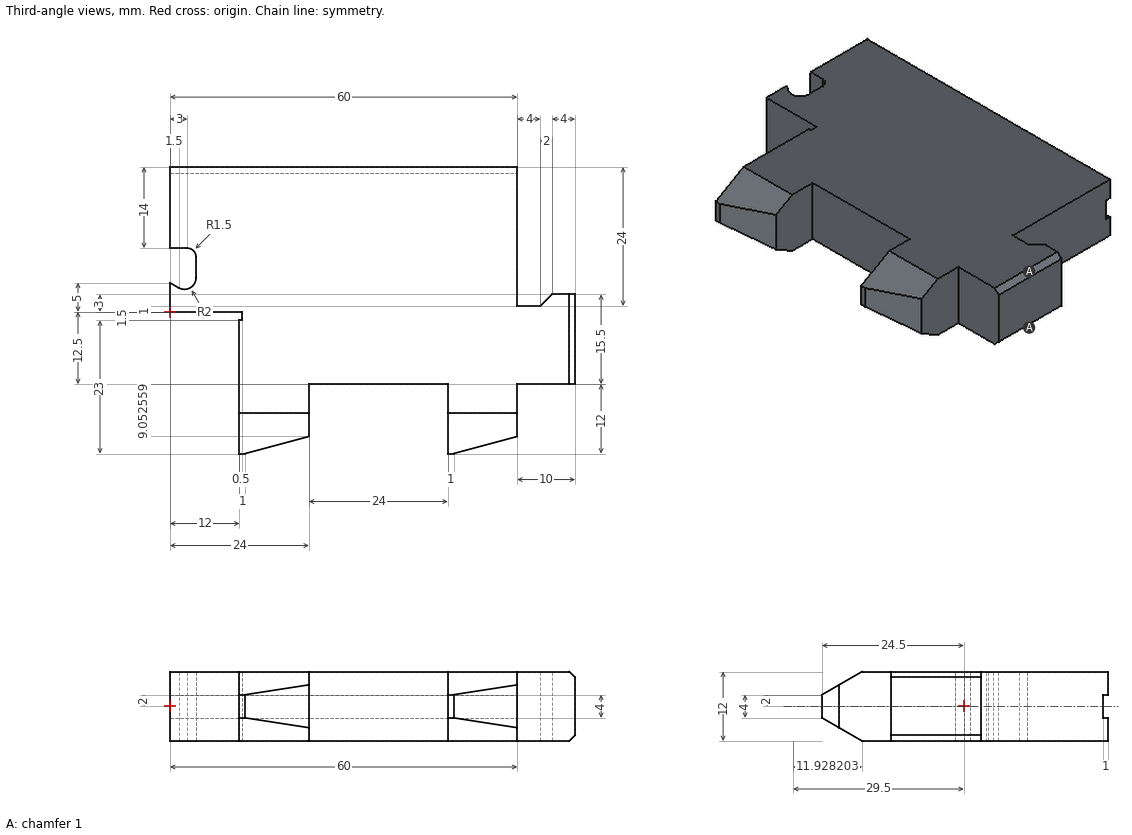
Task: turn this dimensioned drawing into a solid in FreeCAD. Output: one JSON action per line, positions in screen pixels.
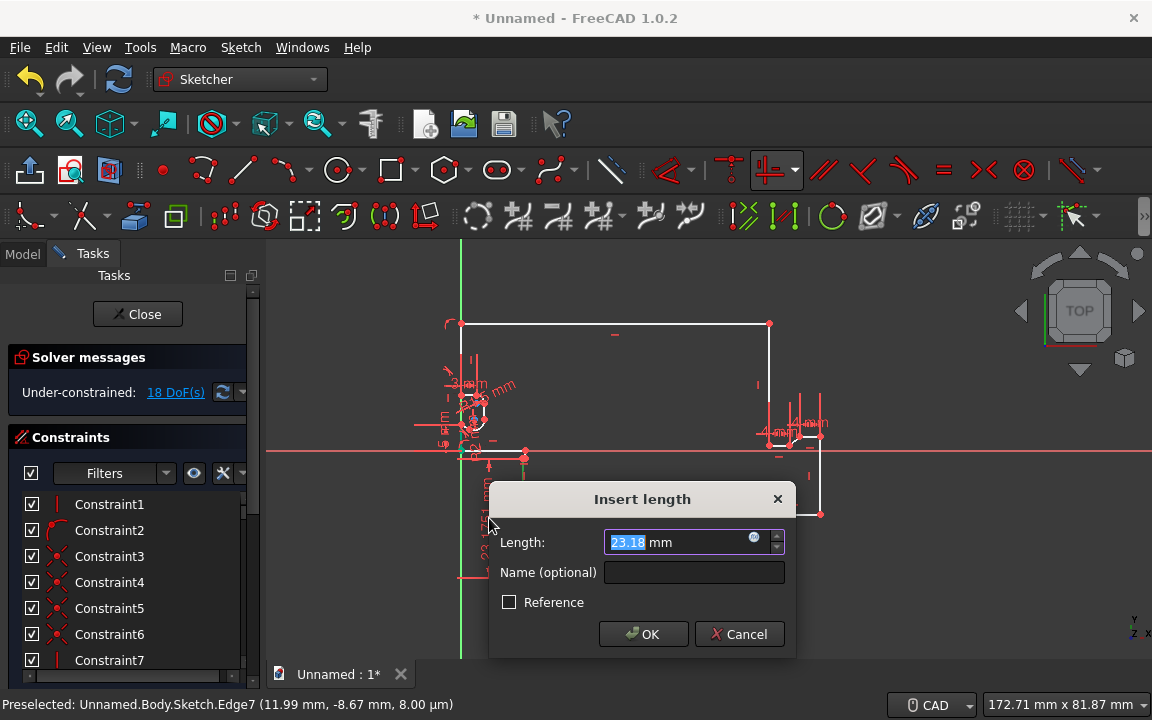
{"action": "type", "text": "23"}
{"action": "key", "text": "Return"}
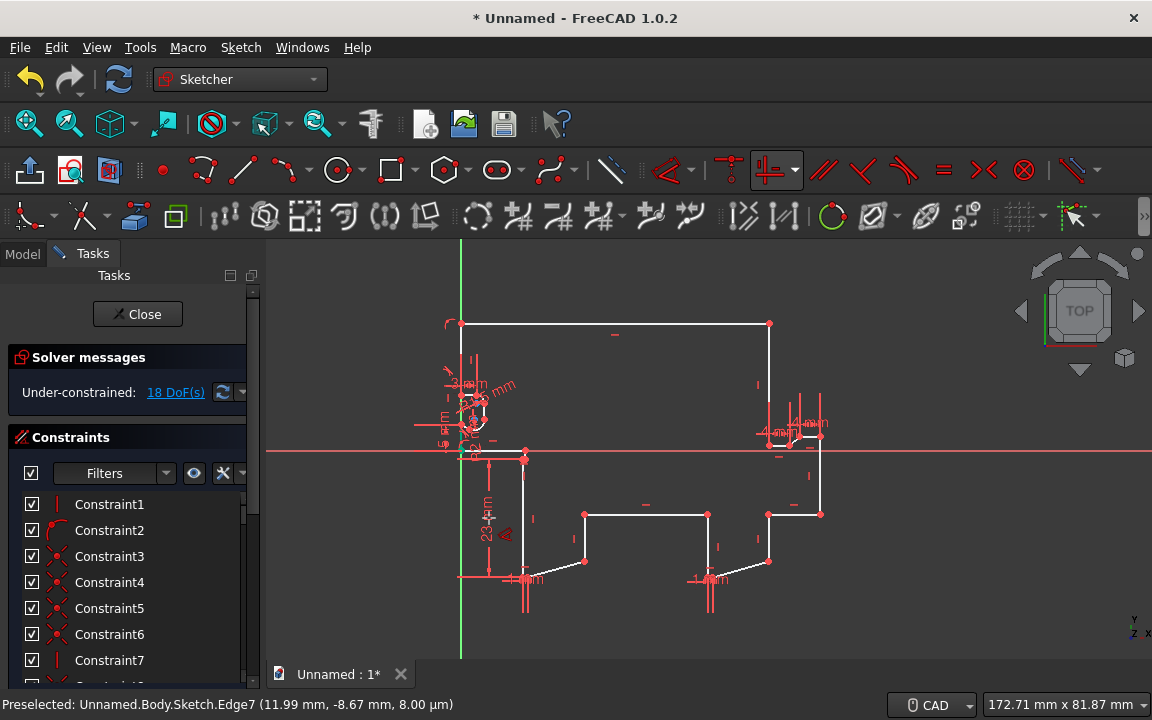
{"action": "left_click", "coordinate": [621, 515]}
{"action": "left_click", "coordinate": [646, 549]}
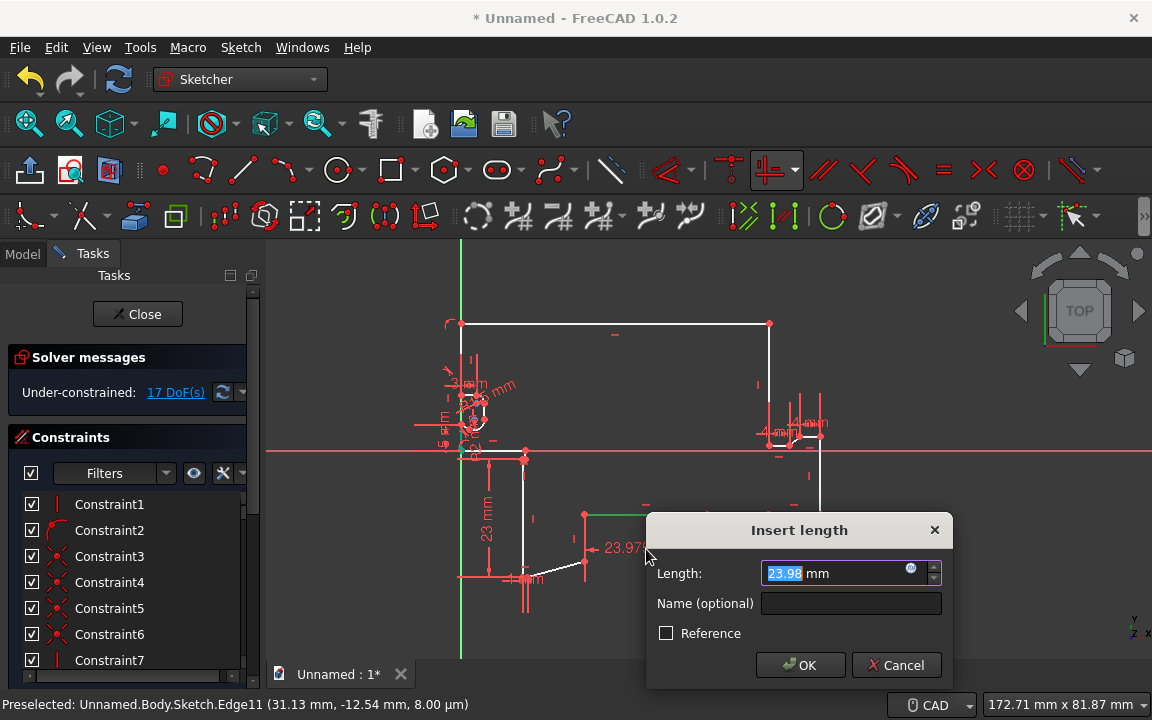
{"action": "type", "text": "24"}
{"action": "key", "text": "Return"}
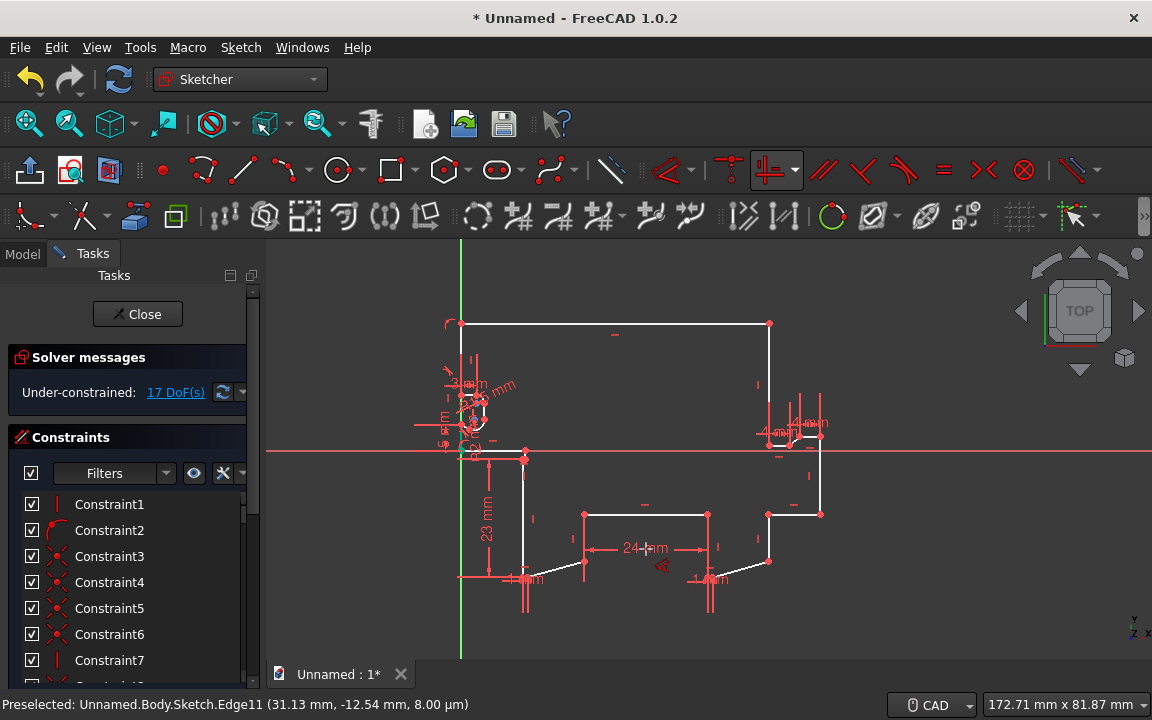
{"action": "left_click", "coordinate": [708, 534]}
{"action": "left_click", "coordinate": [742, 546]}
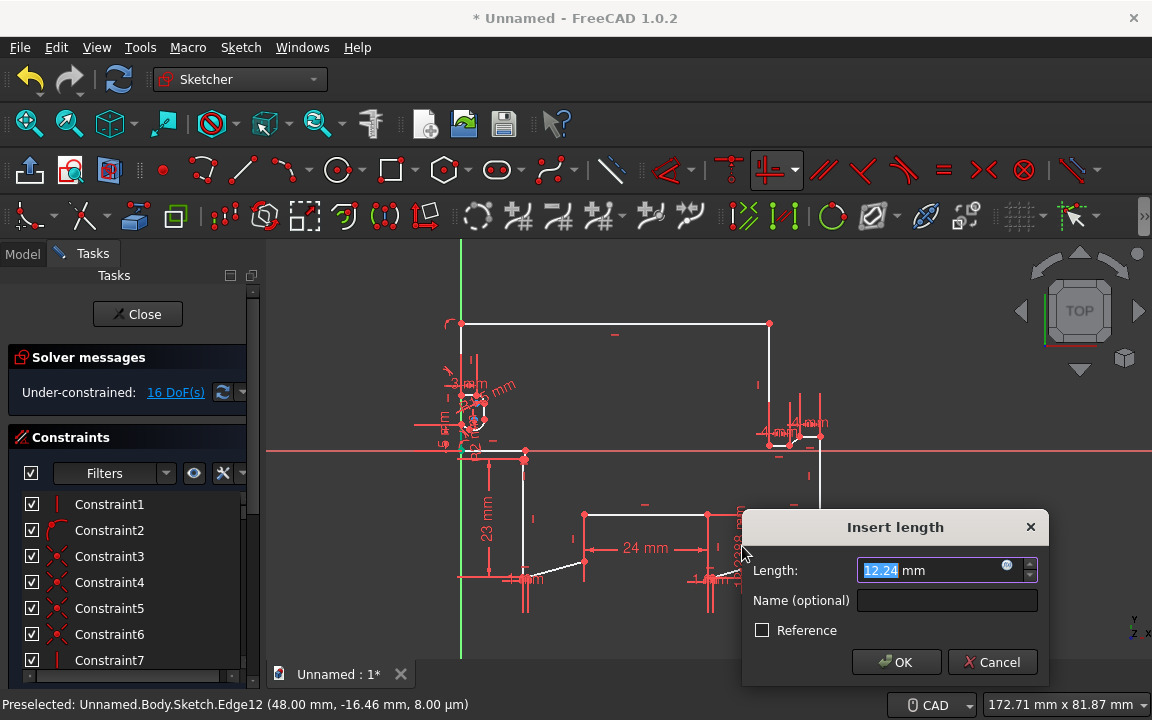
{"action": "type", "text": "12"}
{"action": "key", "text": "Return"}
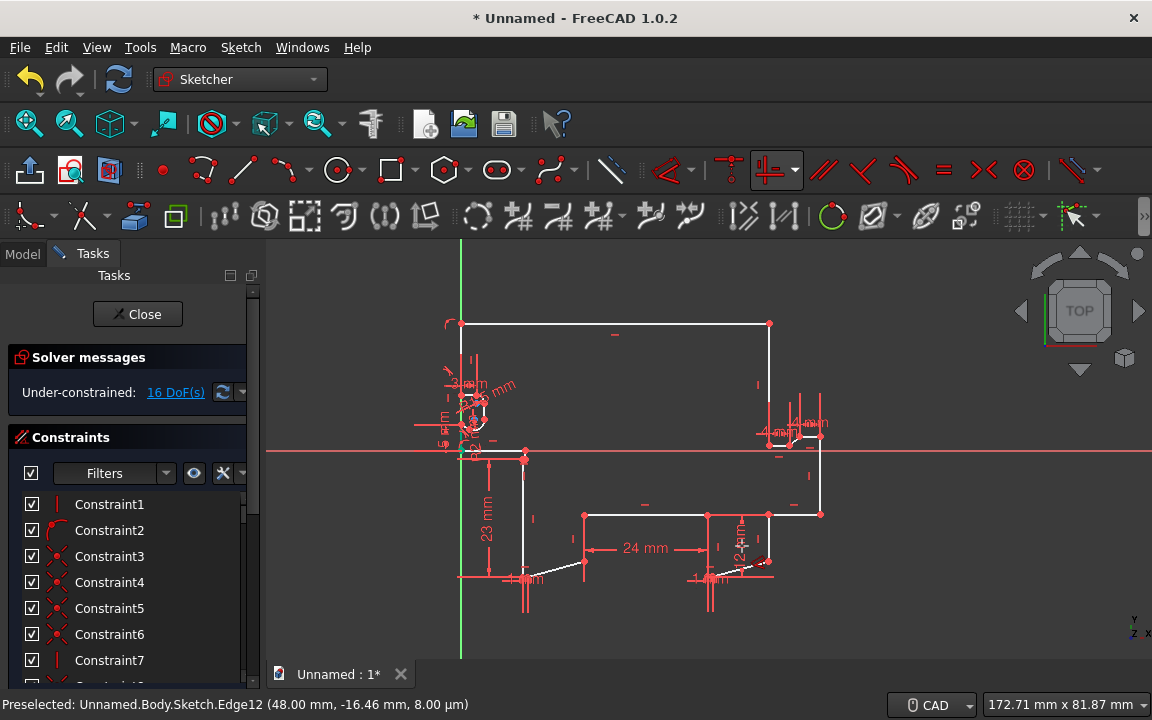
{"action": "left_click", "coordinate": [784, 515]}
{"action": "left_click", "coordinate": [813, 549]}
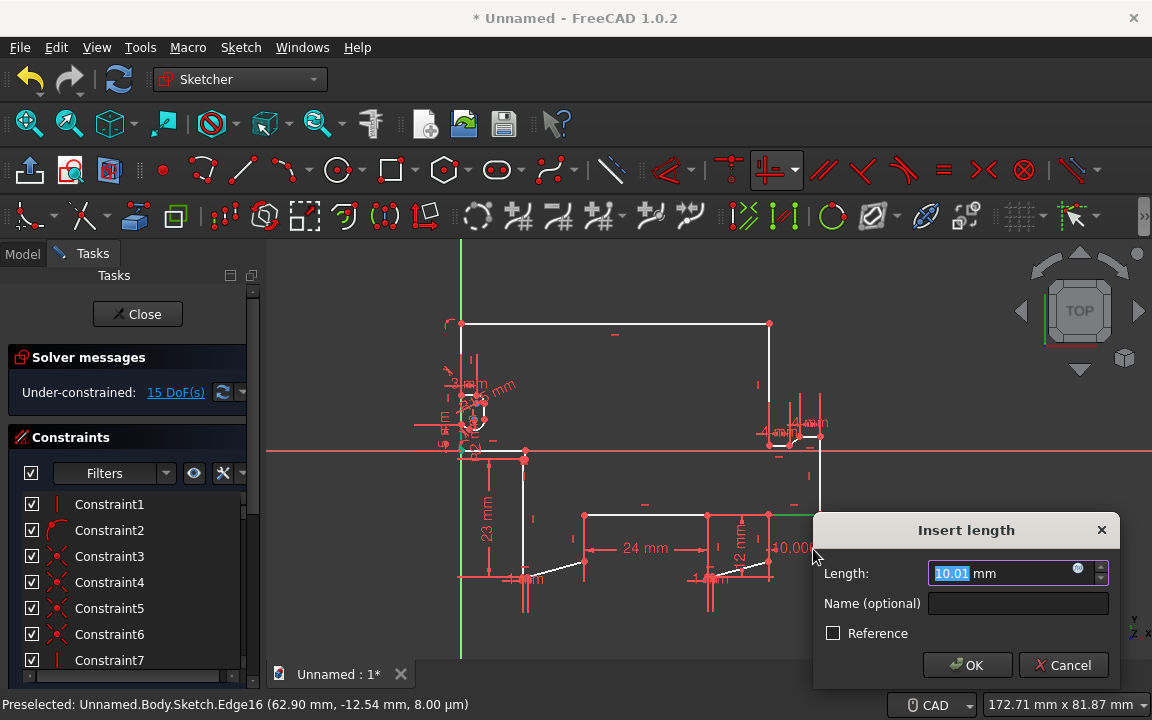
{"action": "type", "text": "10"}
{"action": "key", "text": "Return"}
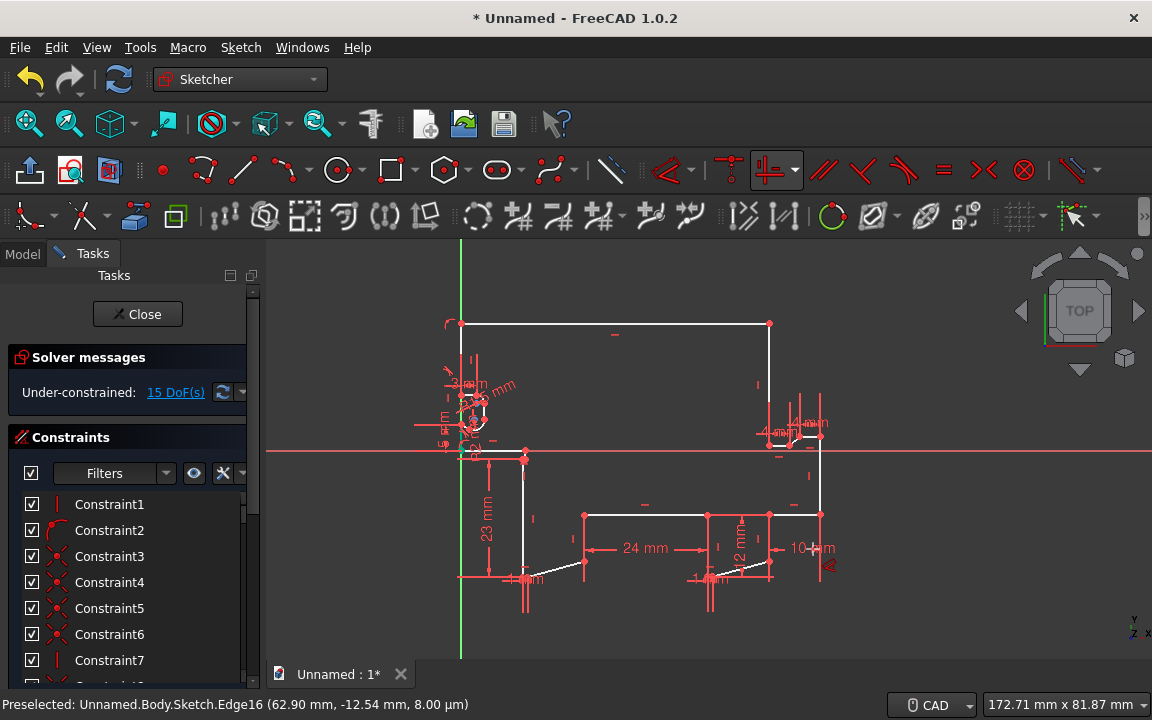
{"action": "left_click", "coordinate": [769, 409]}
{"action": "left_click", "coordinate": [803, 385]}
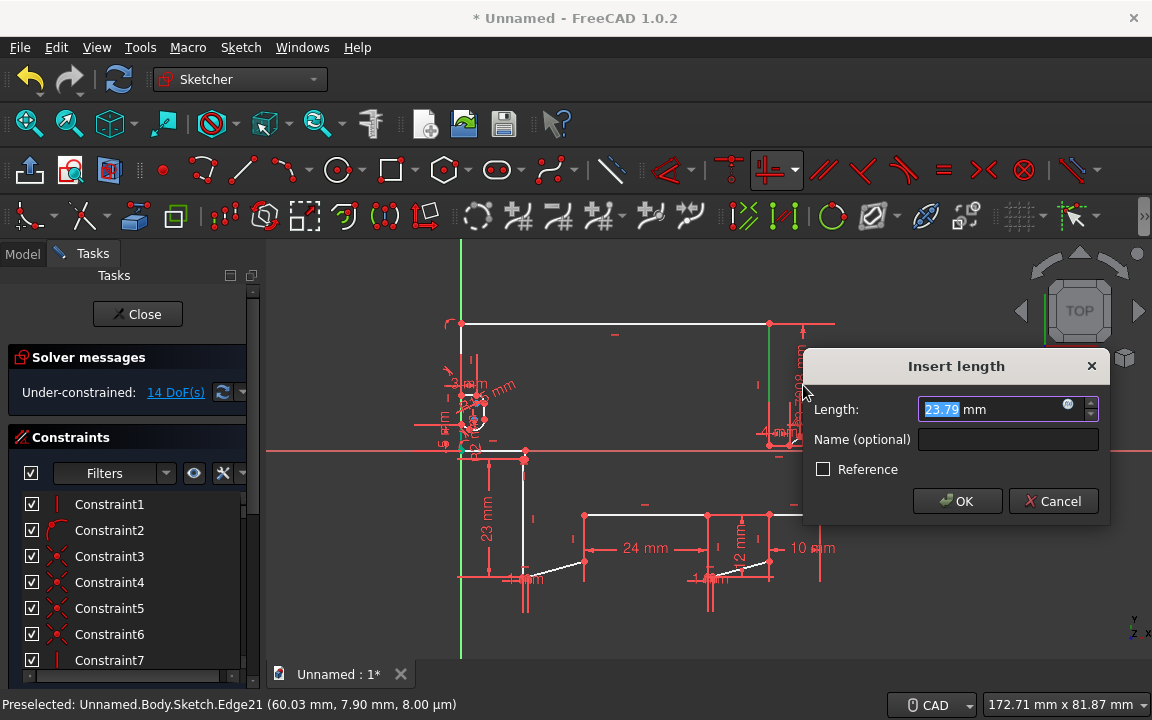
{"action": "type", "text": "24"}
{"action": "key", "text": "Return"}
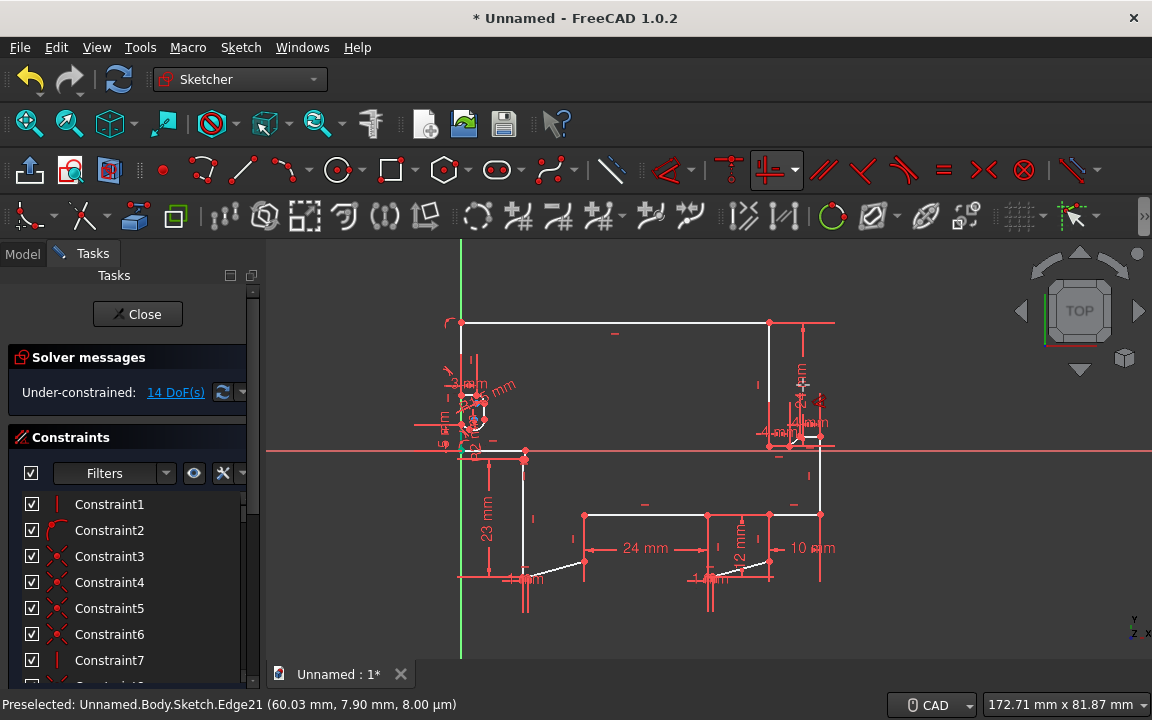
{"action": "left_click", "coordinate": [677, 323]}
{"action": "left_click", "coordinate": [615, 289]}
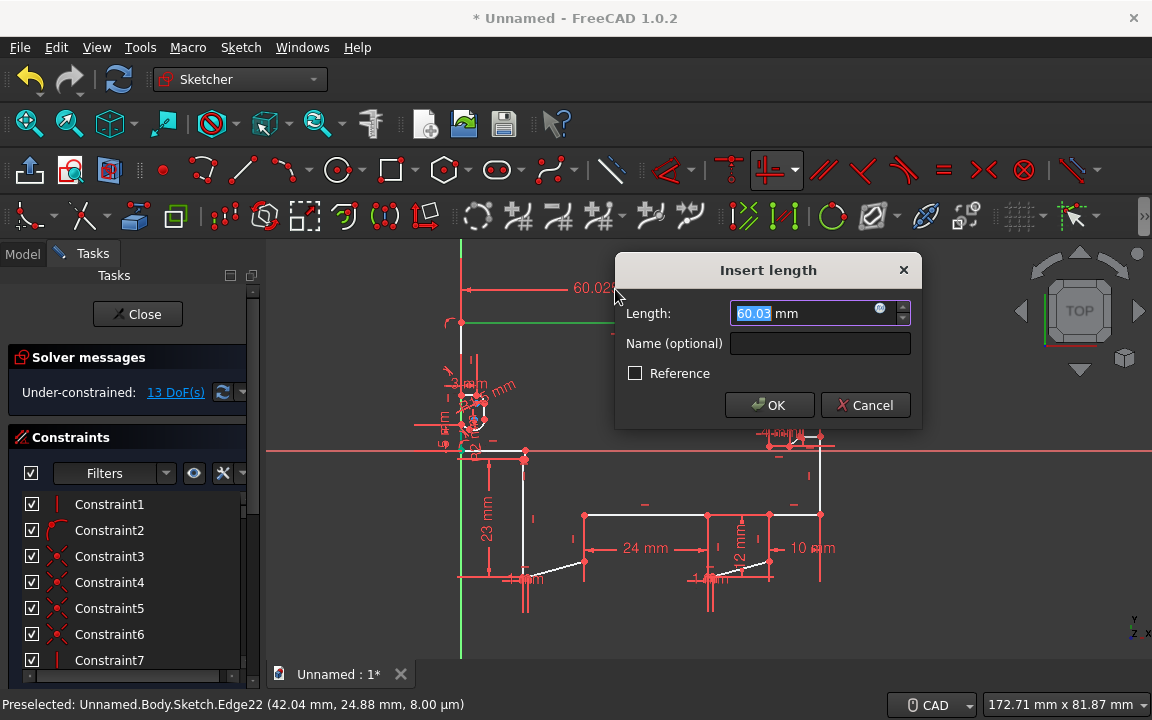
{"action": "type", "text": "60"}
{"action": "key", "text": "Return"}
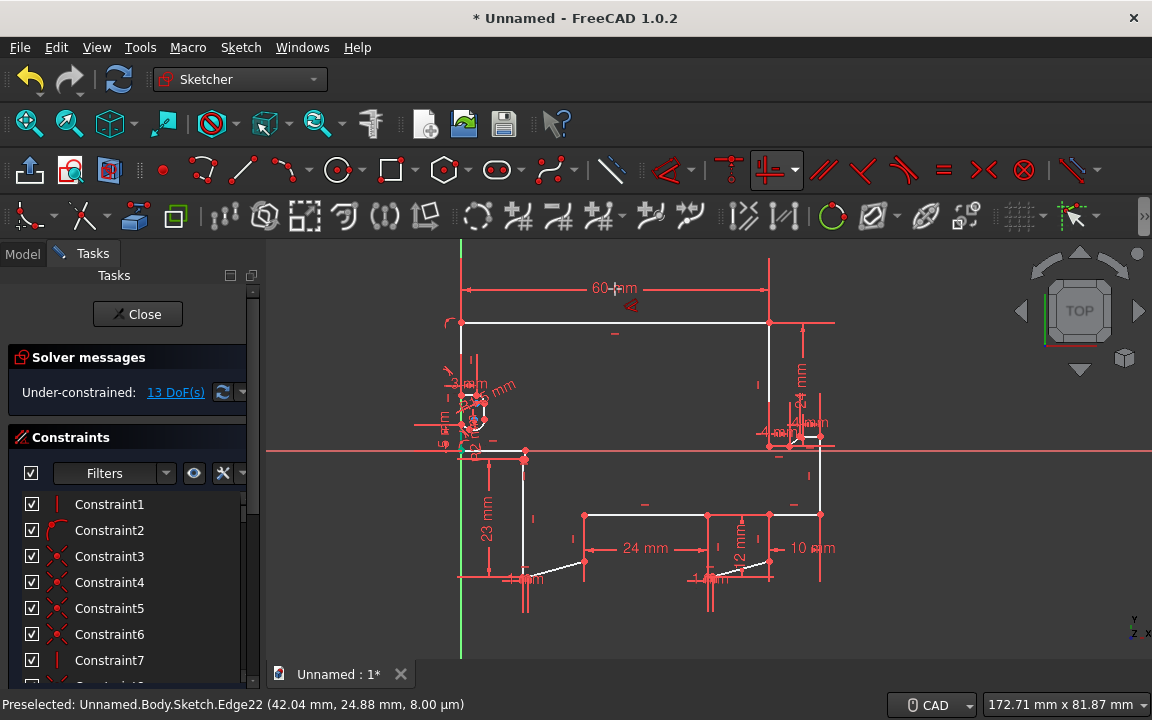
{"action": "left_click", "coordinate": [461, 345]}
{"action": "left_click", "coordinate": [427, 359]}